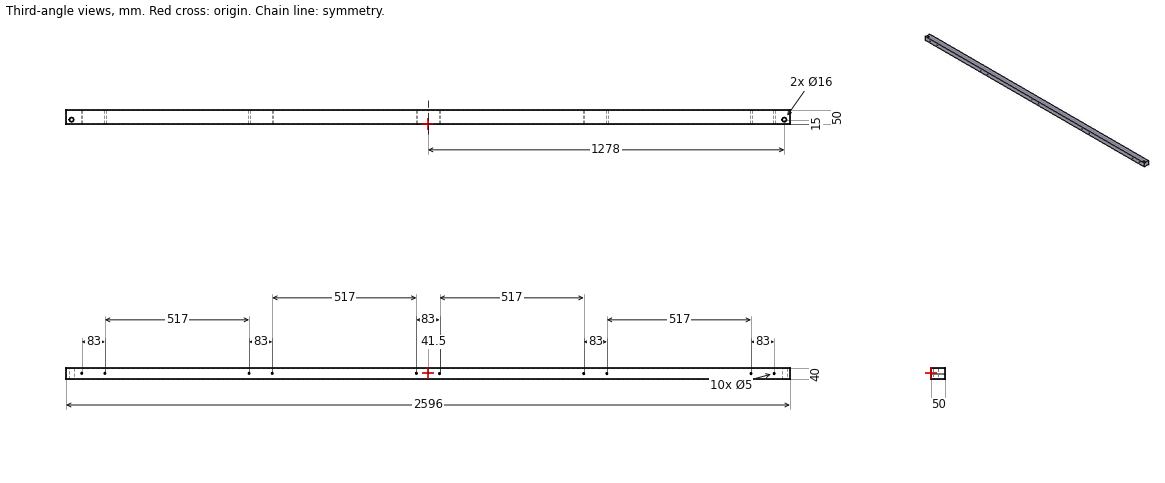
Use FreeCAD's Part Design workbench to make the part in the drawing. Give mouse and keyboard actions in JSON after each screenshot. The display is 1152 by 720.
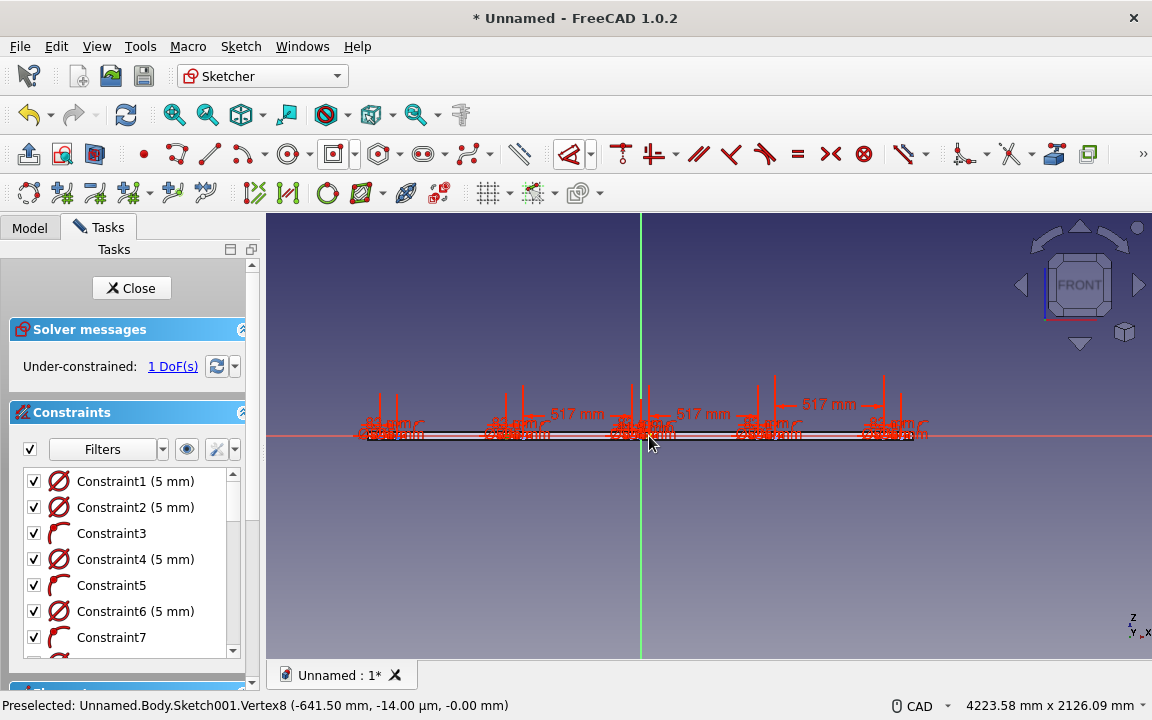
{"action": "left_click", "coordinate": [397, 436]}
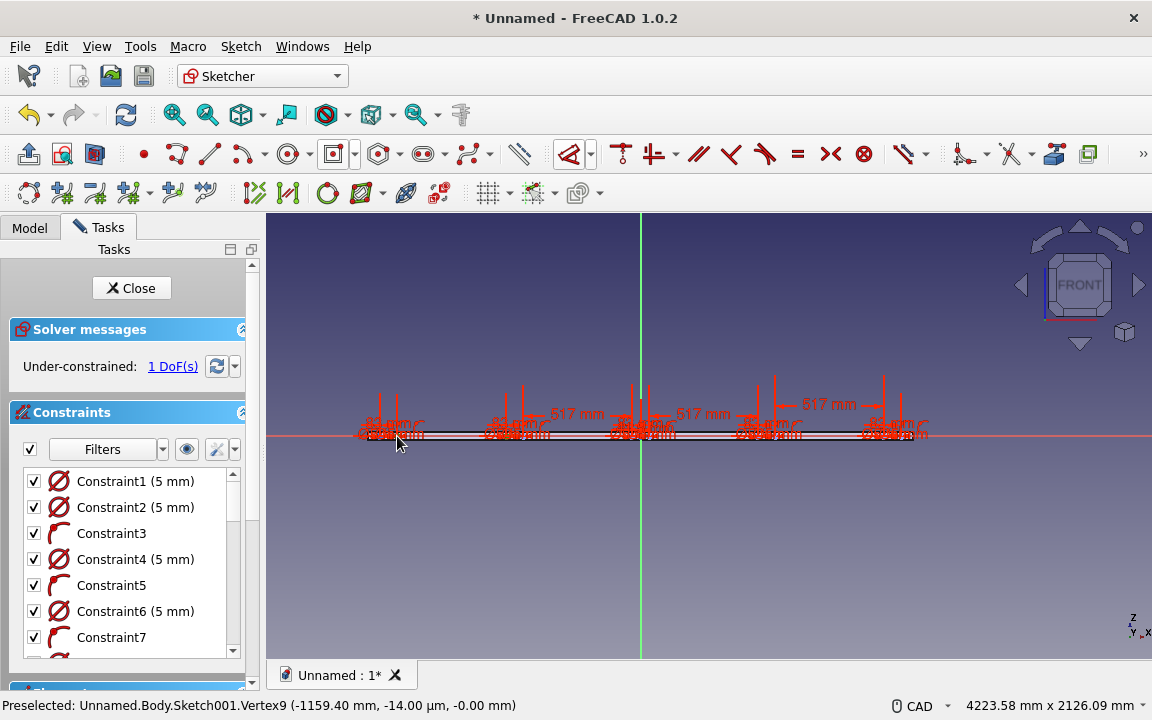
{"action": "left_click", "coordinate": [590, 154]}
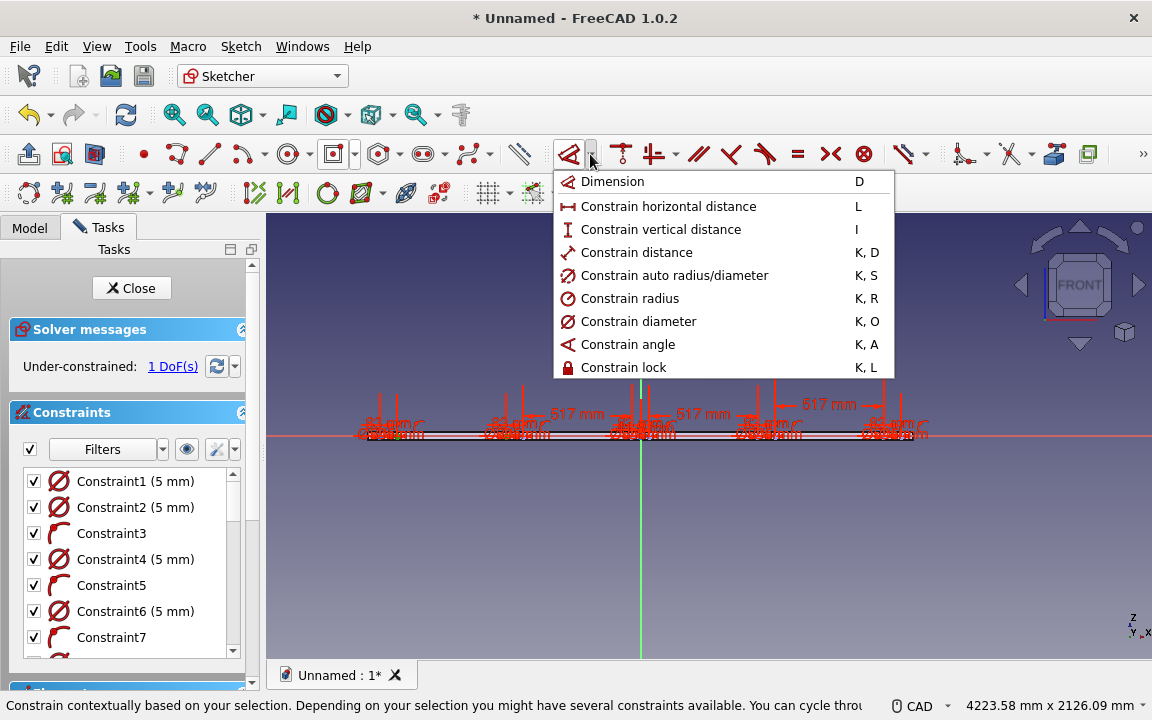
{"action": "left_click", "coordinate": [724, 206]}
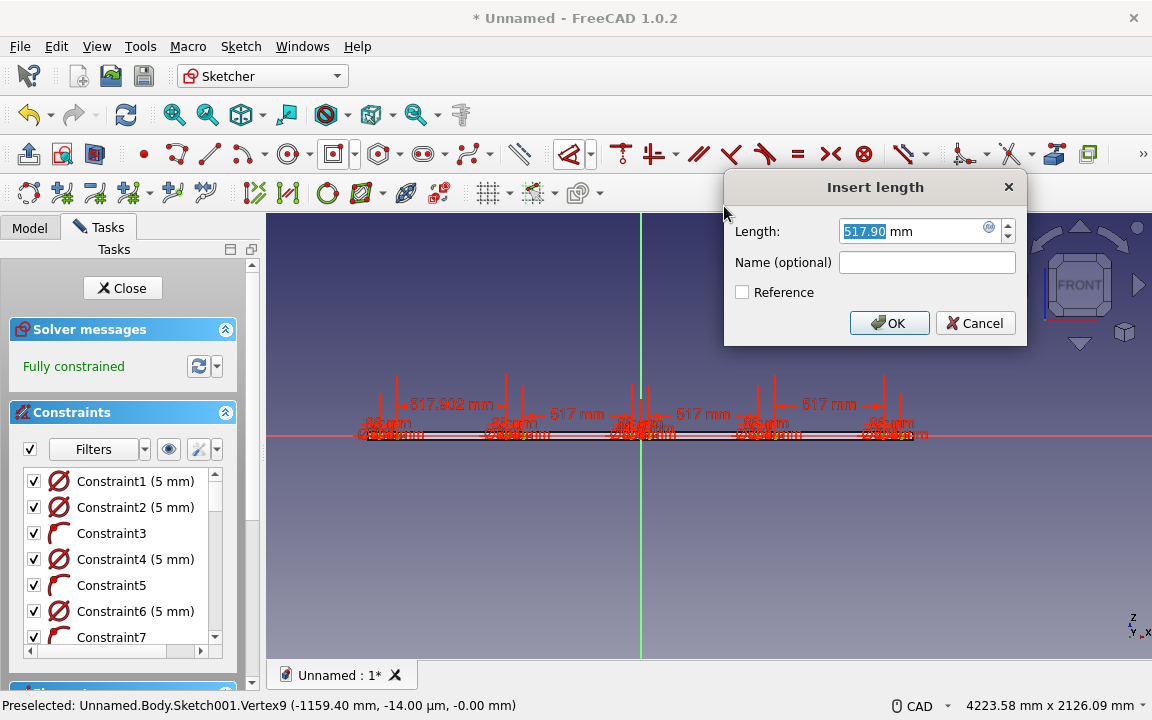
{"action": "type", "text": "517"}
{"action": "key", "text": "Return"}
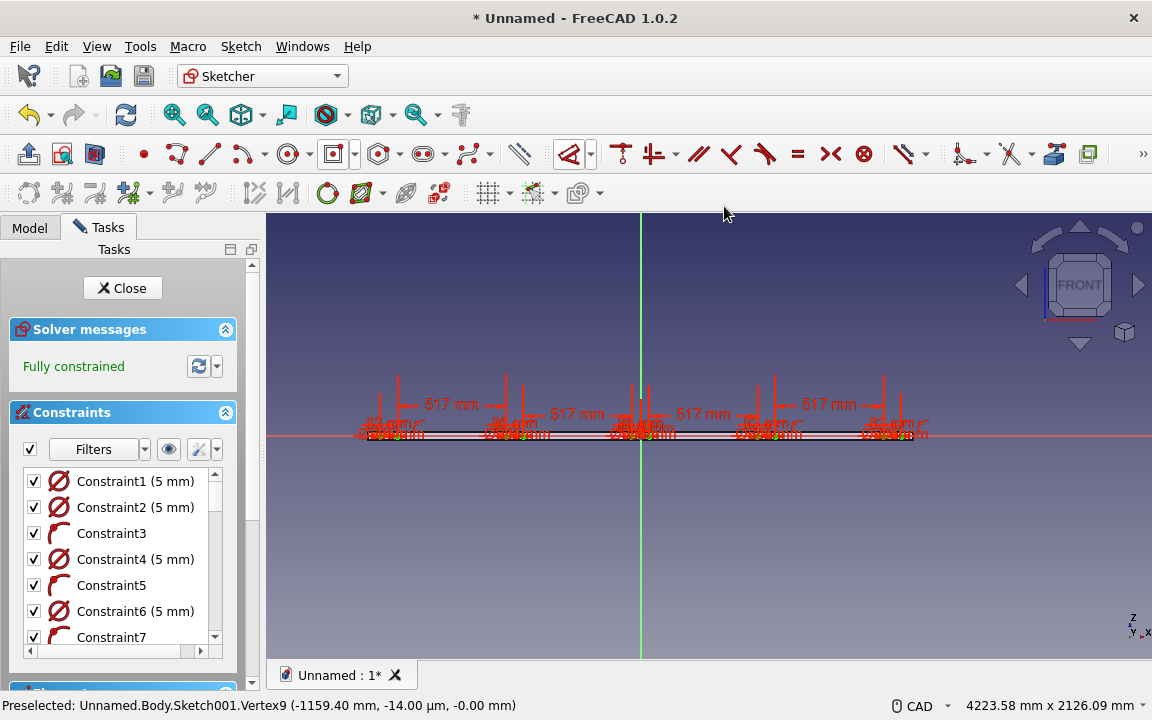
{"action": "left_click", "coordinate": [123, 288]}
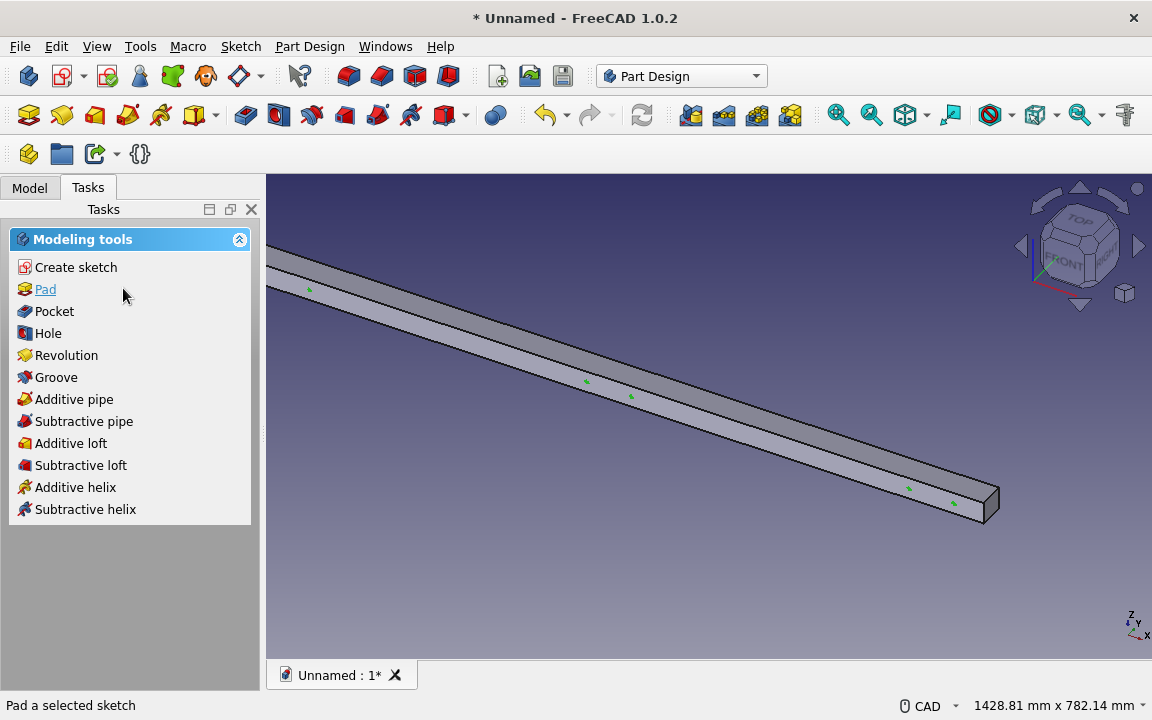
{"action": "left_click", "coordinate": [246, 116]}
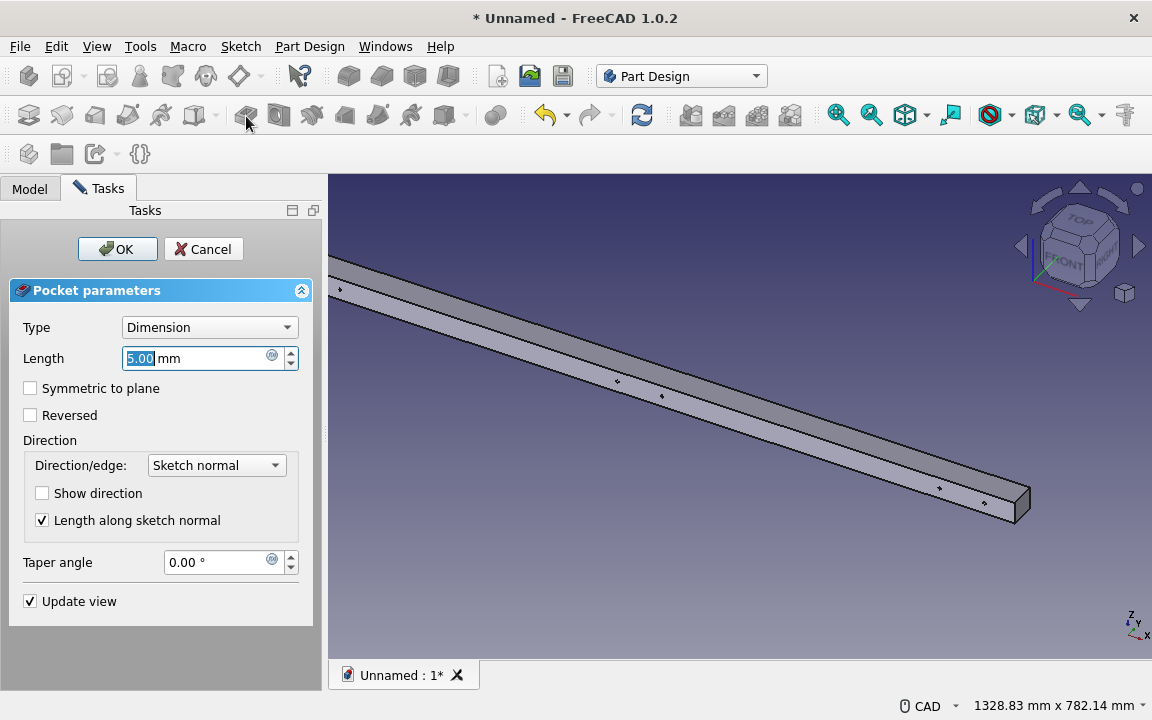
{"action": "type", "text": "50"}
{"action": "key", "text": "Tab"}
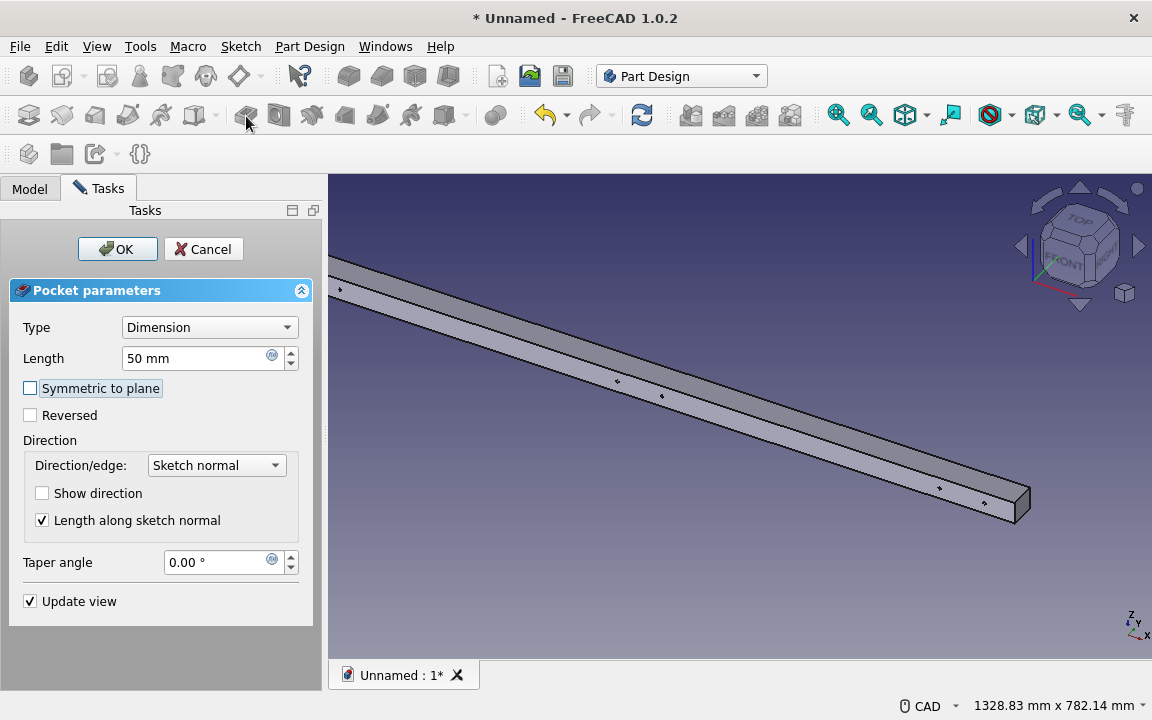
{"action": "left_click", "coordinate": [118, 249]}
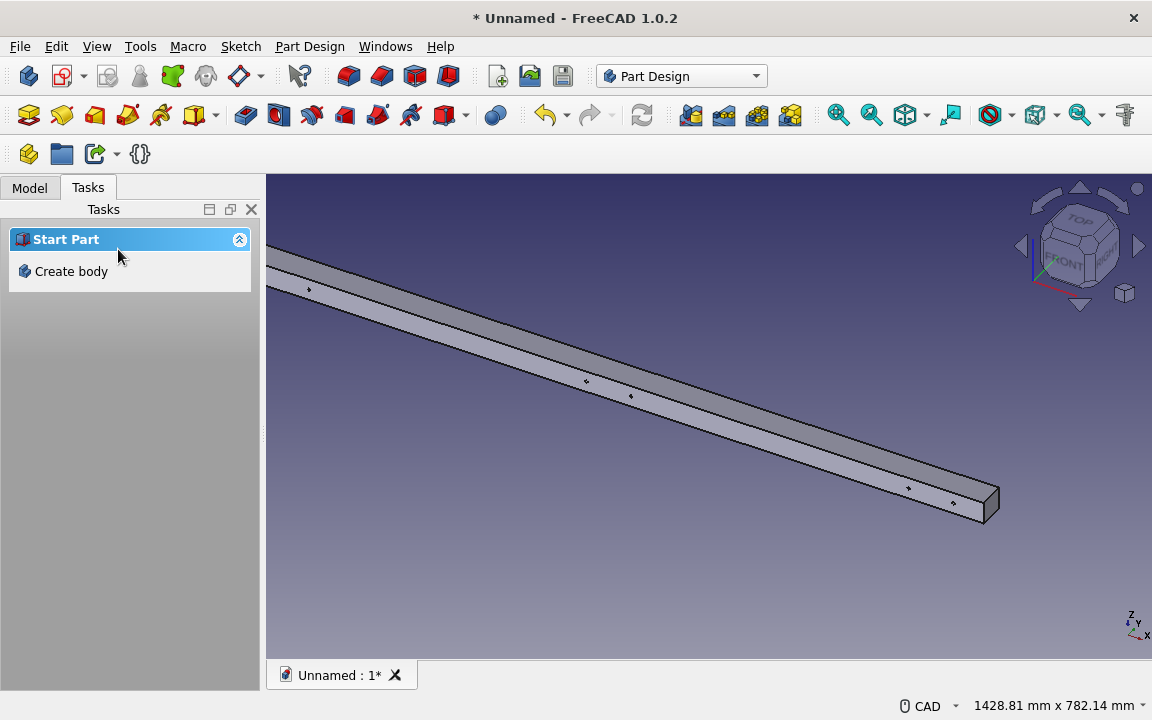
{"action": "left_click", "coordinate": [839, 116]}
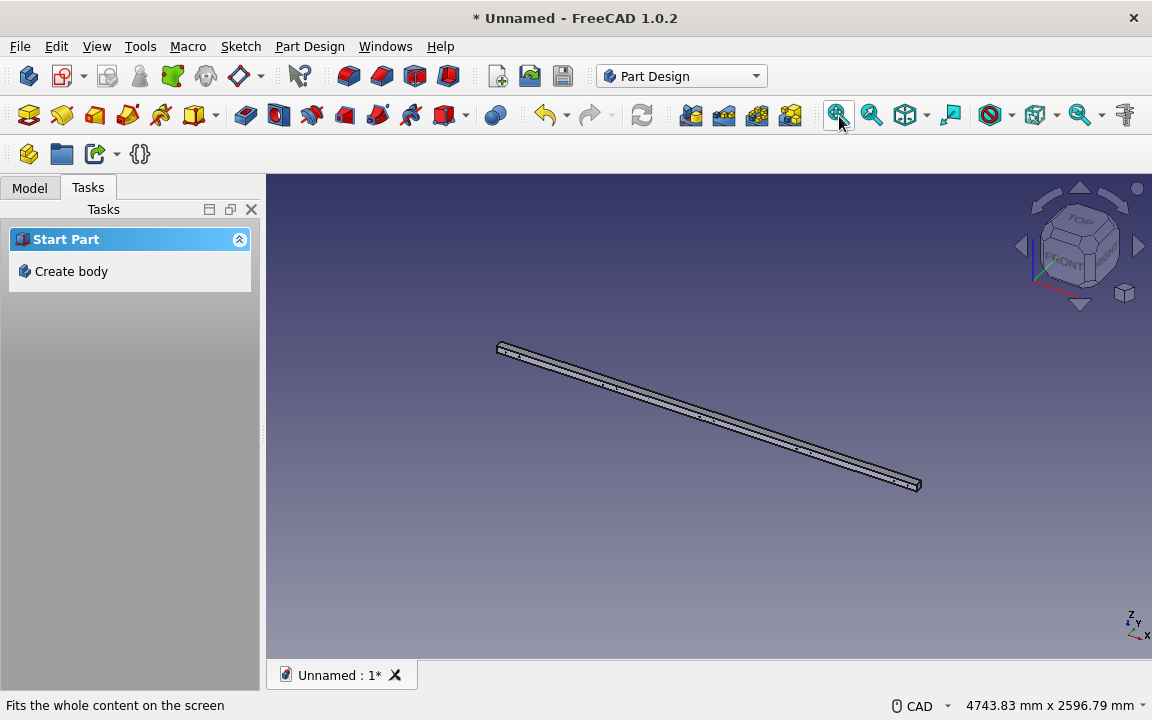
{"action": "key", "text": "5"}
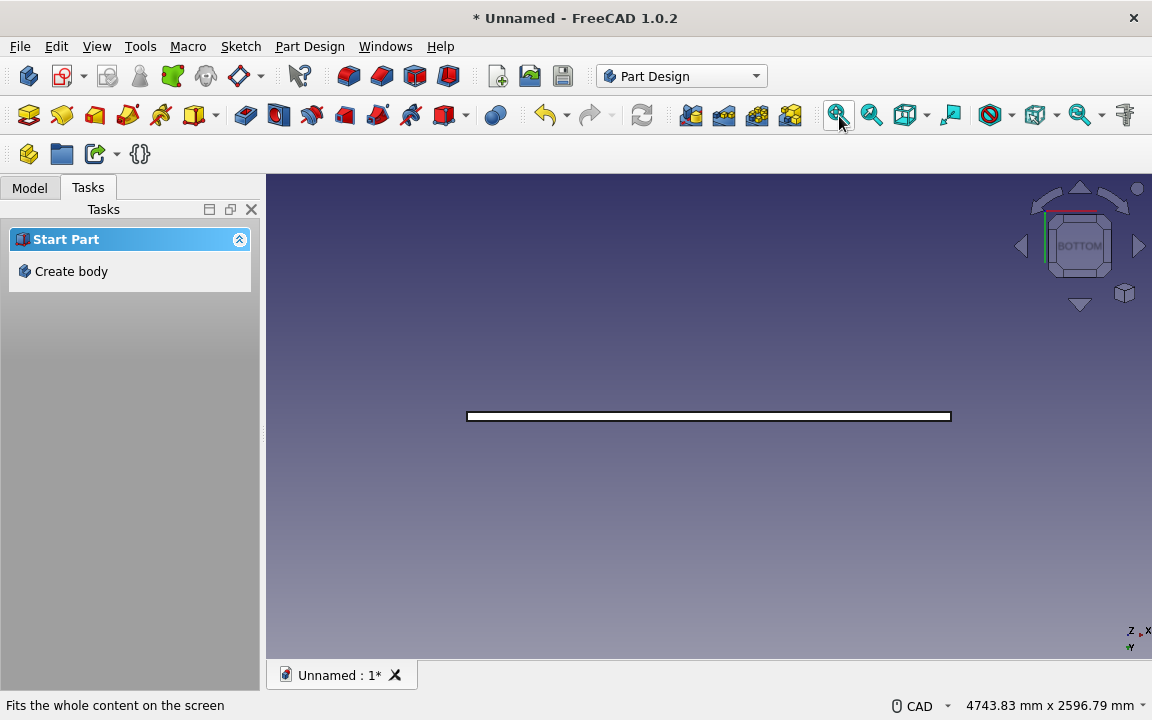
{"action": "scroll", "coordinate": [917, 415], "scroll_direction": "up", "scroll_amount": 5}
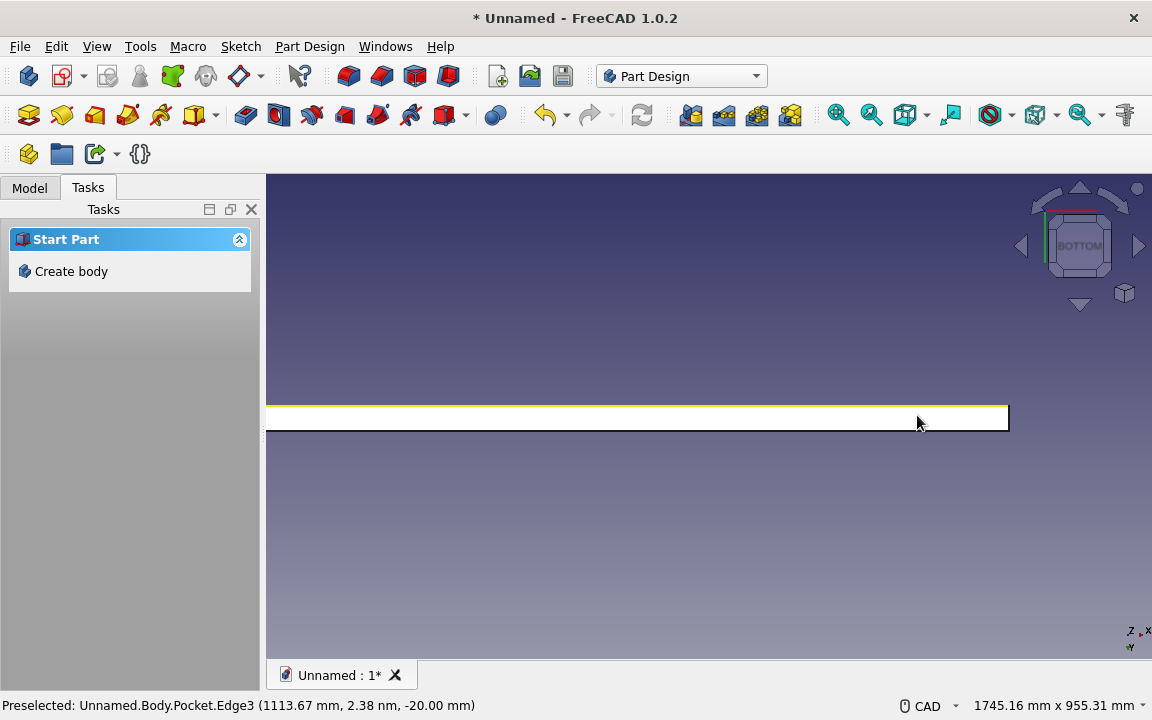
{"action": "left_click", "coordinate": [915, 417]}